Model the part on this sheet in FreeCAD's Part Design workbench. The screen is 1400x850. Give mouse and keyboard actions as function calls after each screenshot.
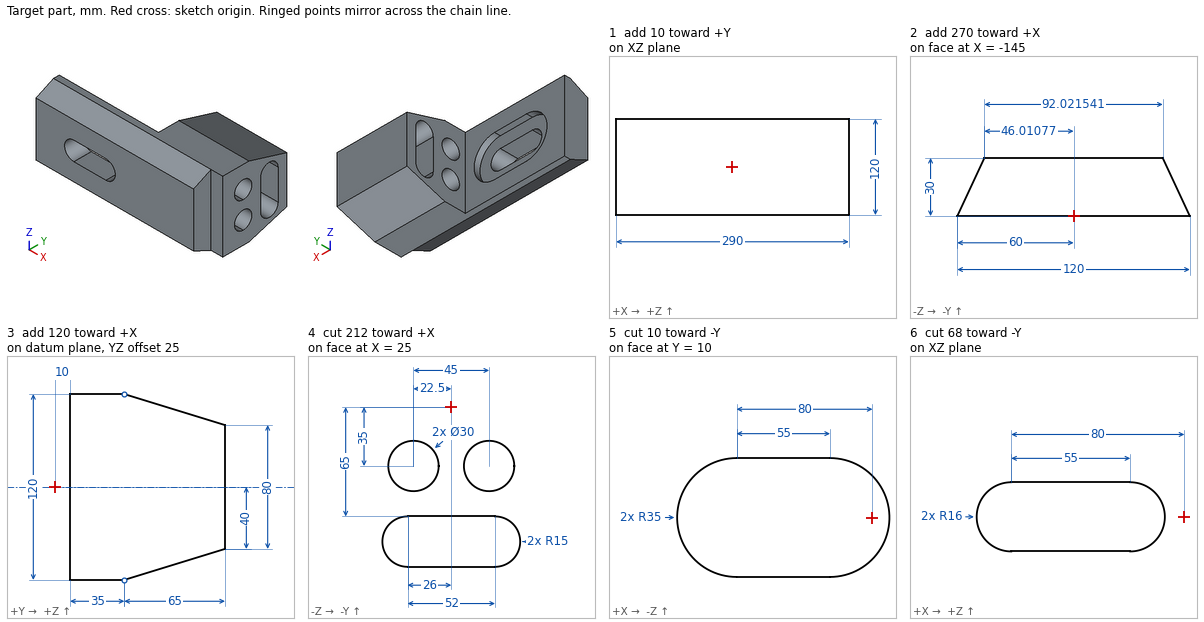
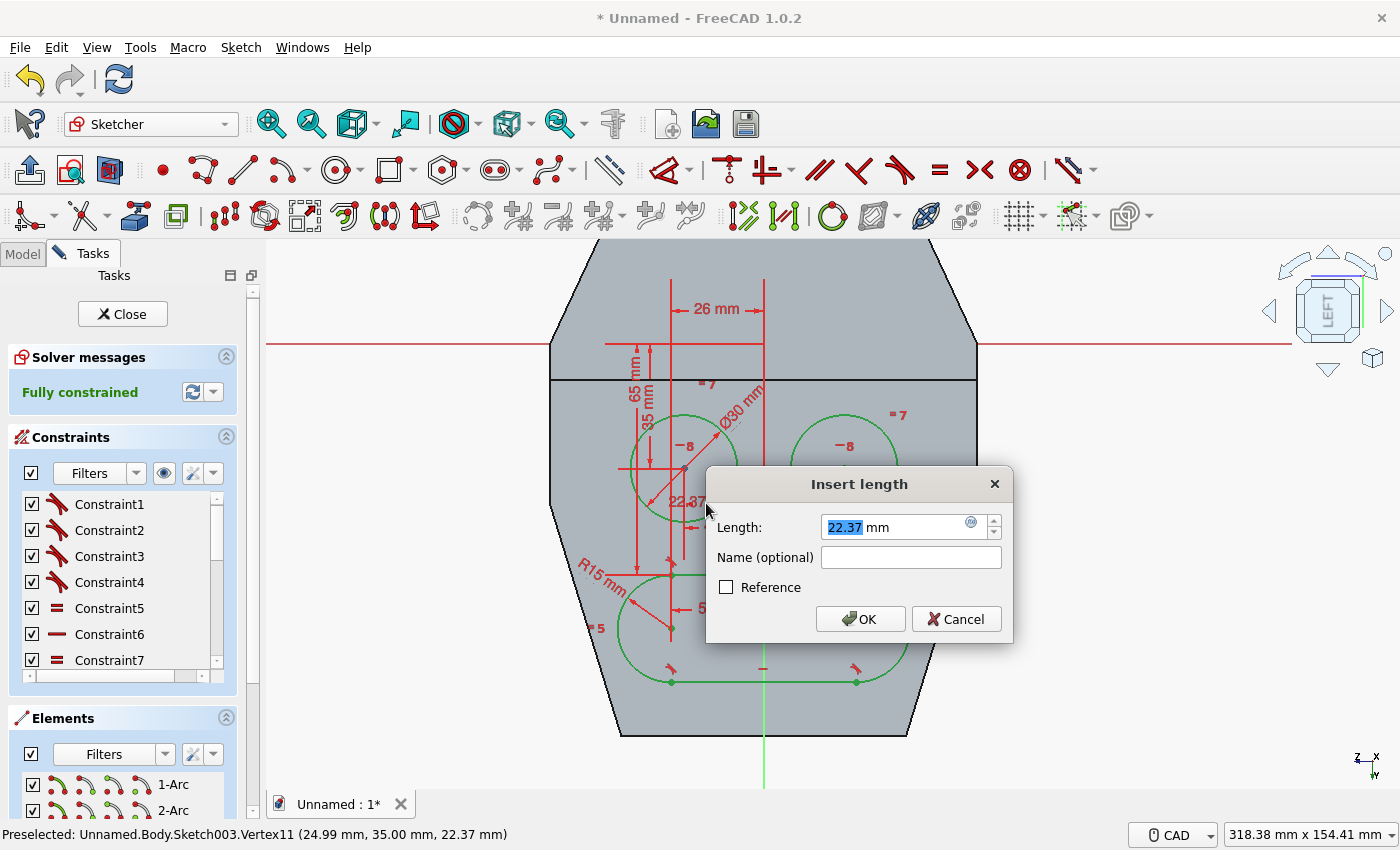
text(22.5)
key(Return)
key(Escape)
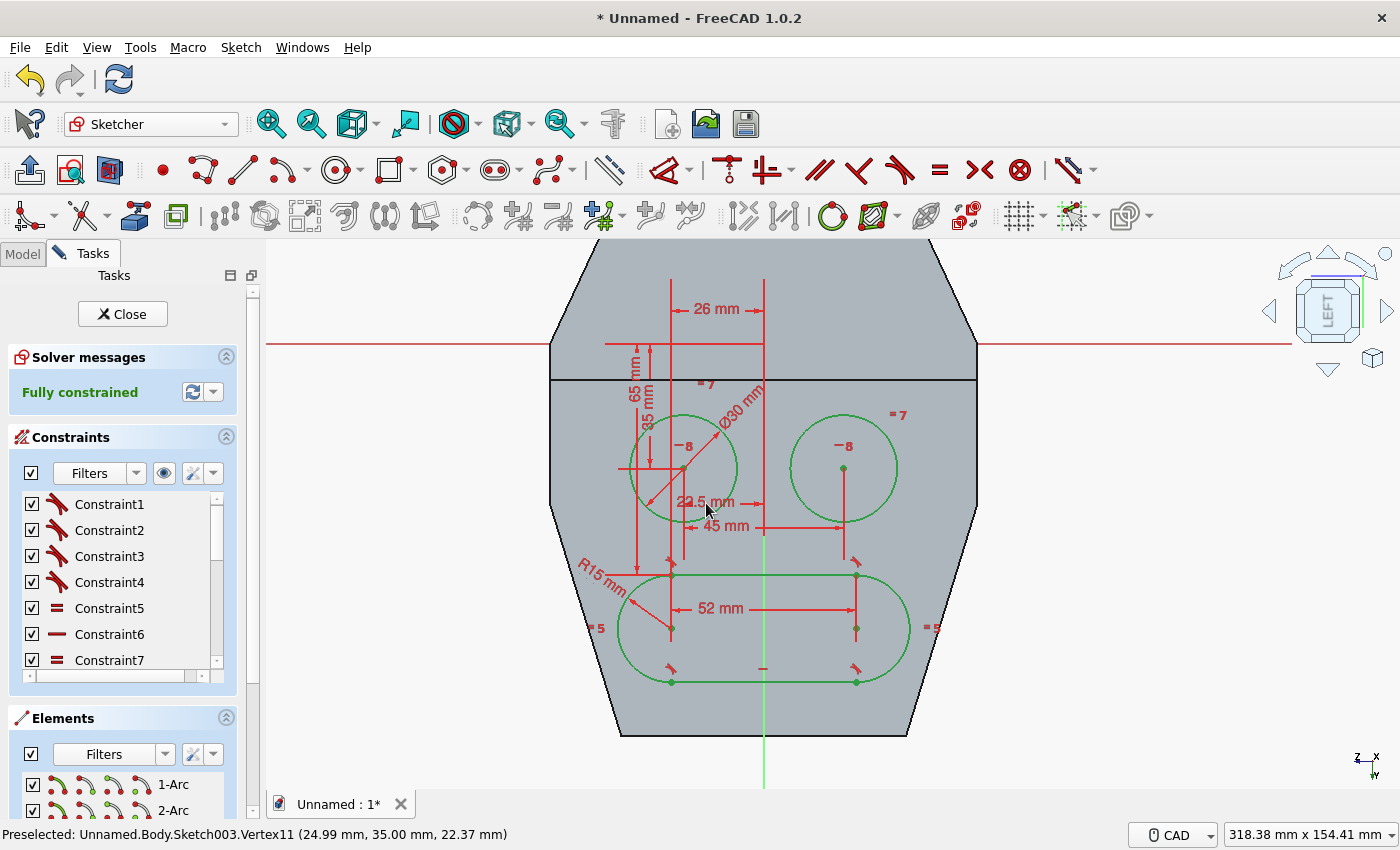
click(123, 314)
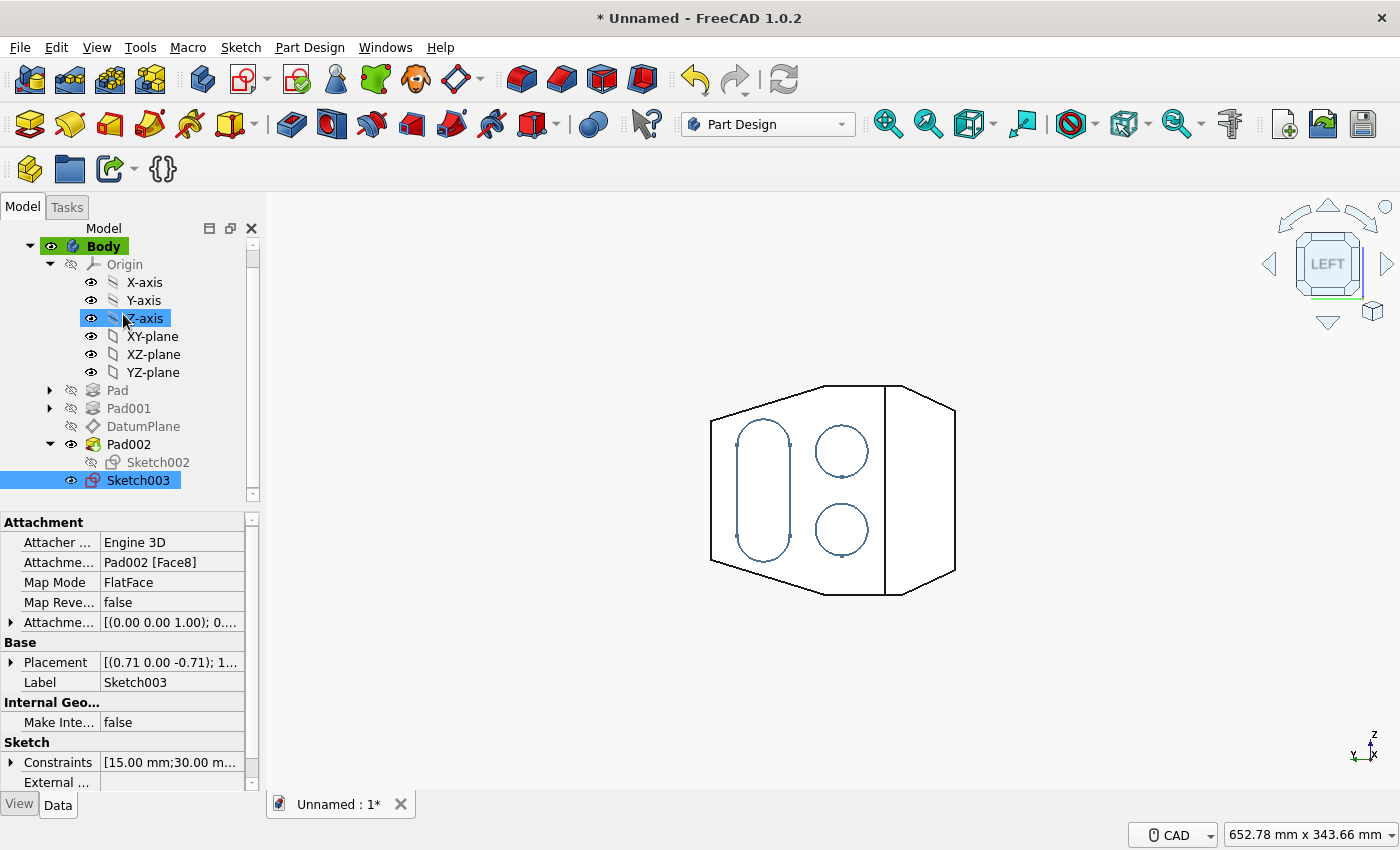
click(292, 124)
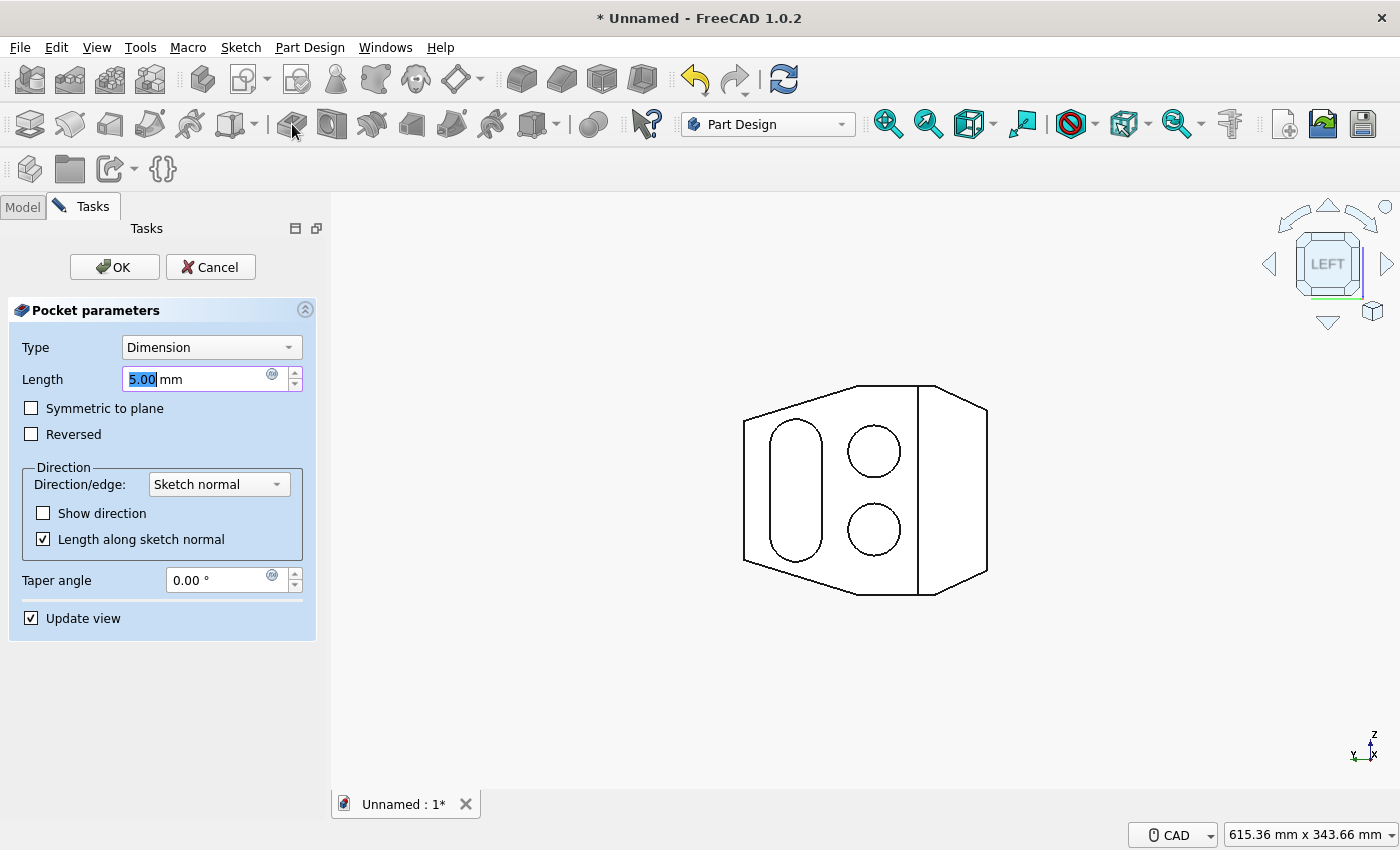
text(212)
key(Tab)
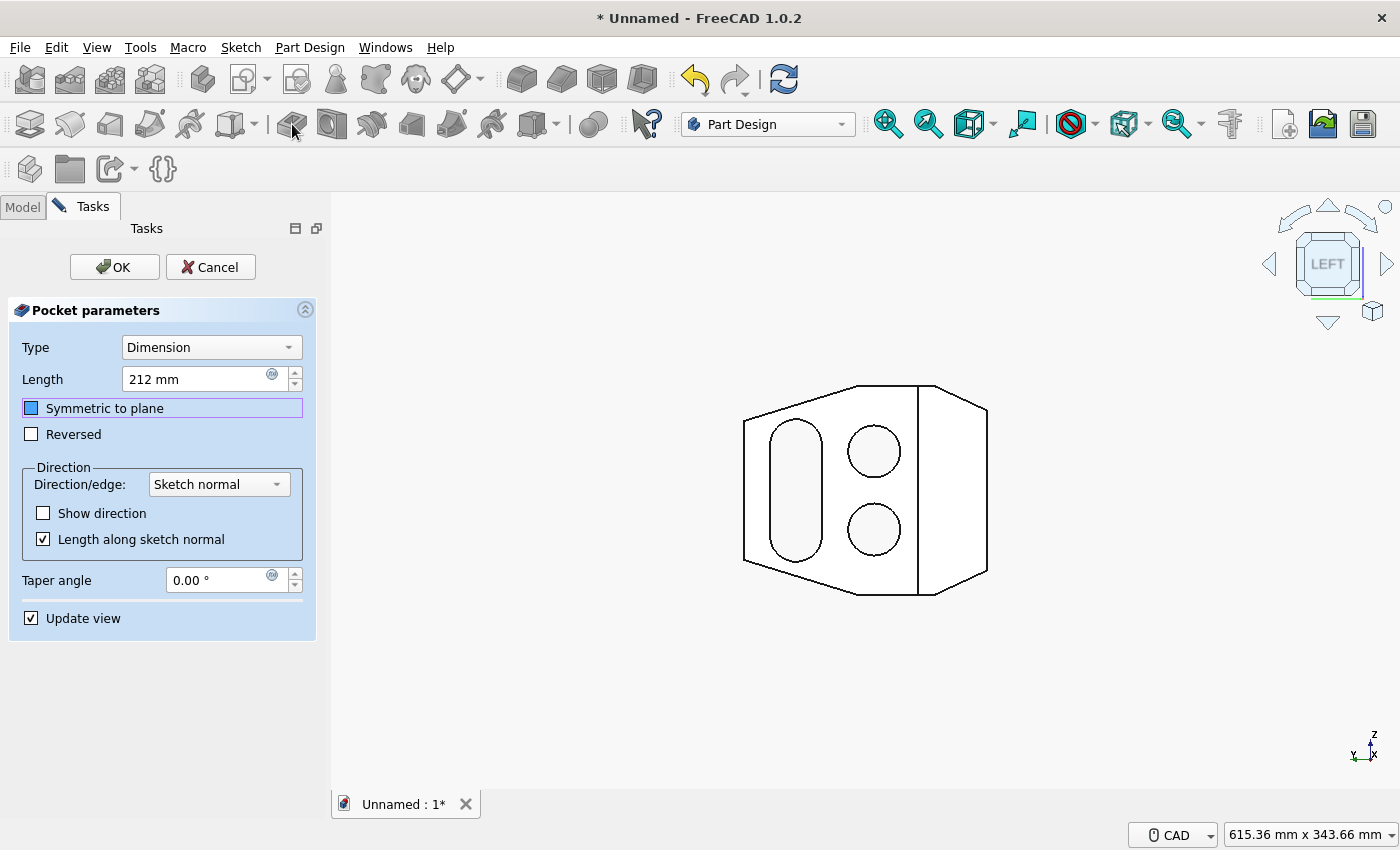
click(115, 267)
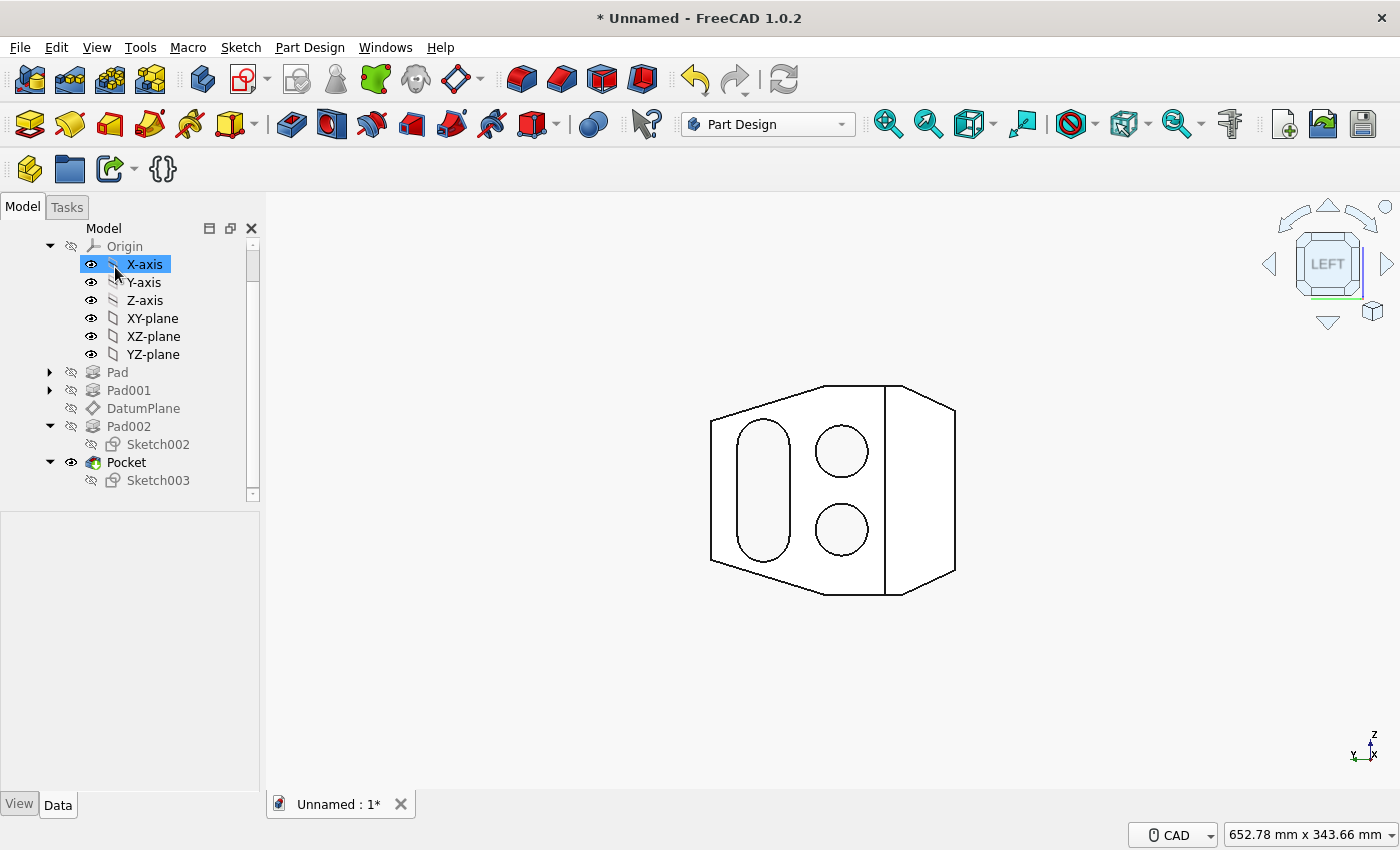
key(v)
key(f)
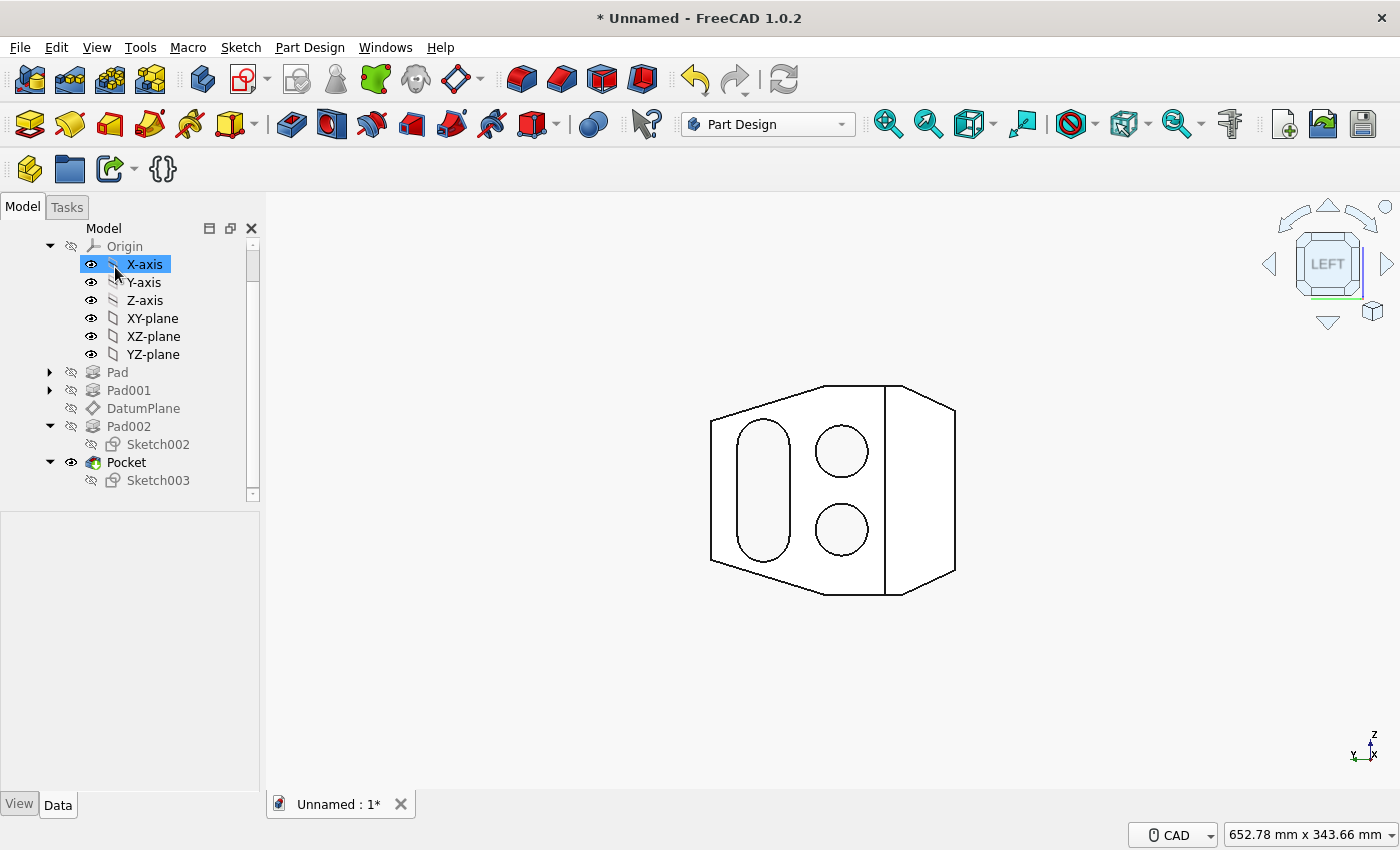
key(4)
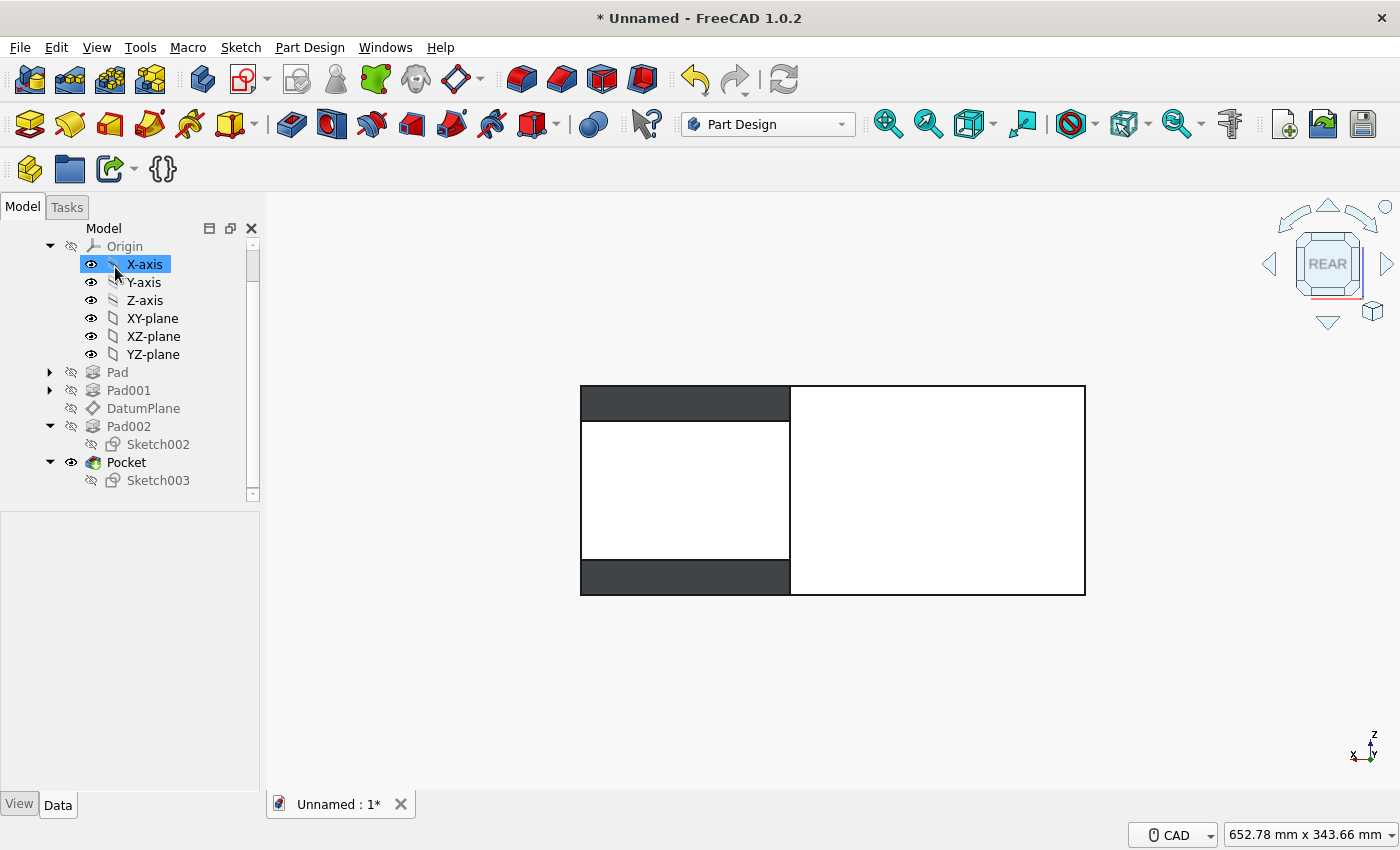
click(890, 124)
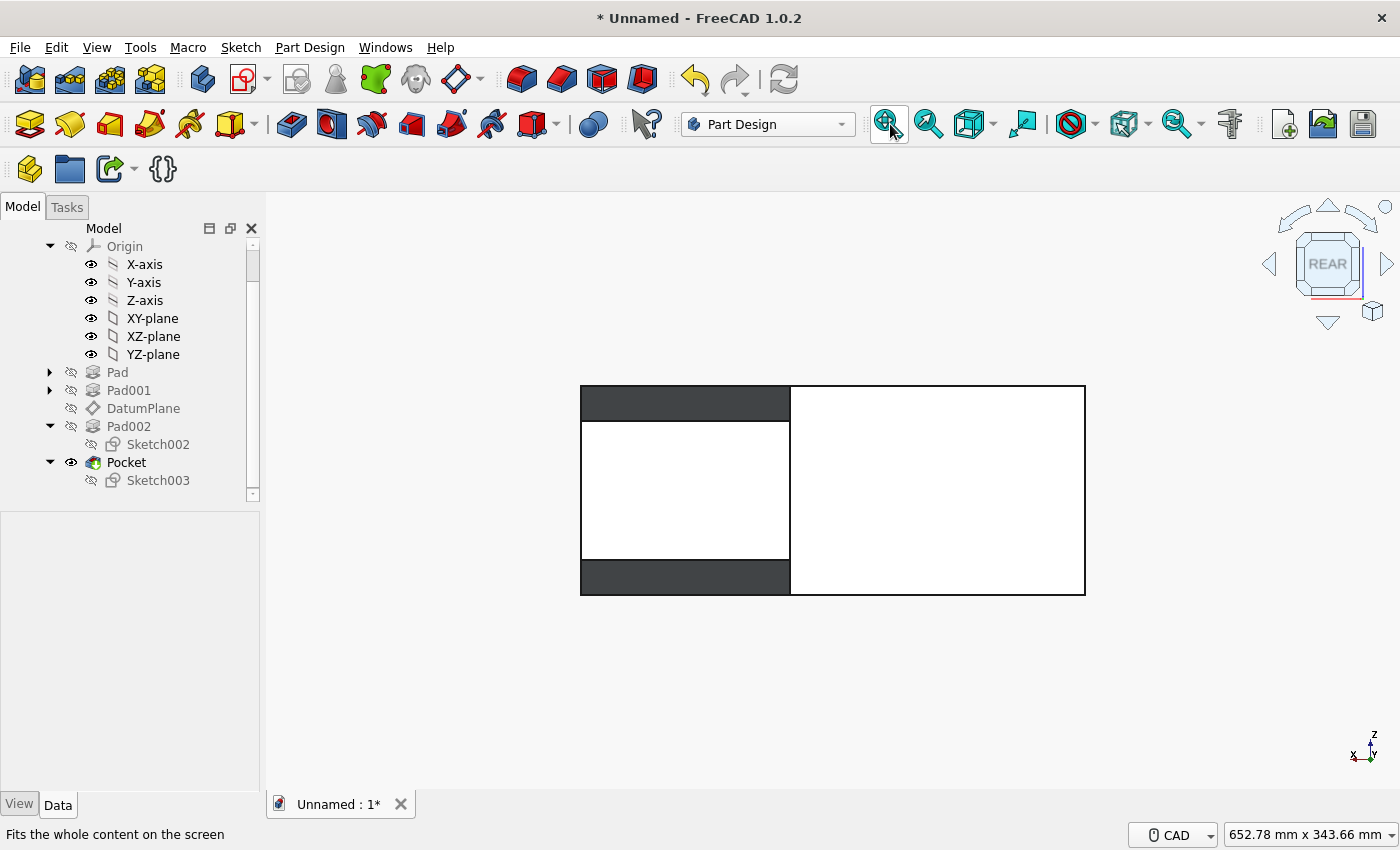
click(895, 490)